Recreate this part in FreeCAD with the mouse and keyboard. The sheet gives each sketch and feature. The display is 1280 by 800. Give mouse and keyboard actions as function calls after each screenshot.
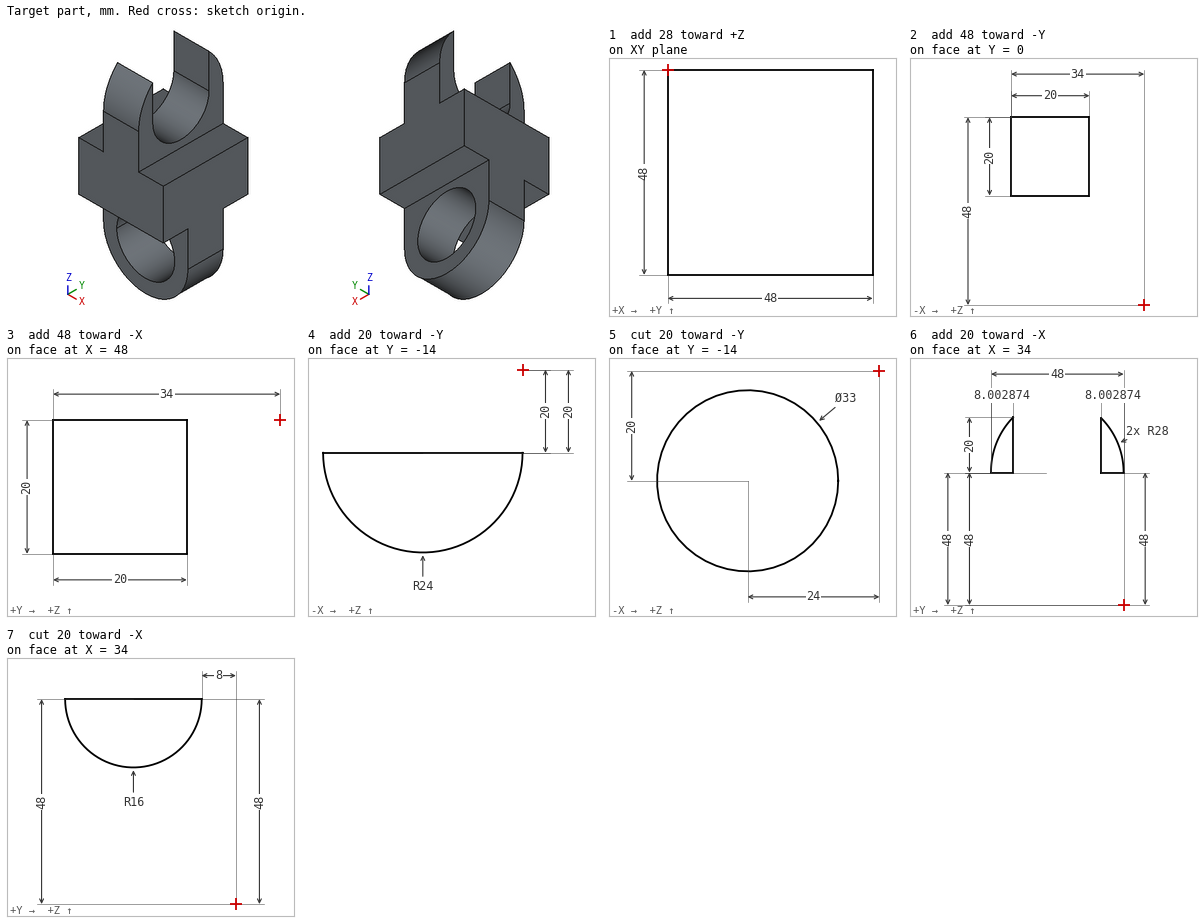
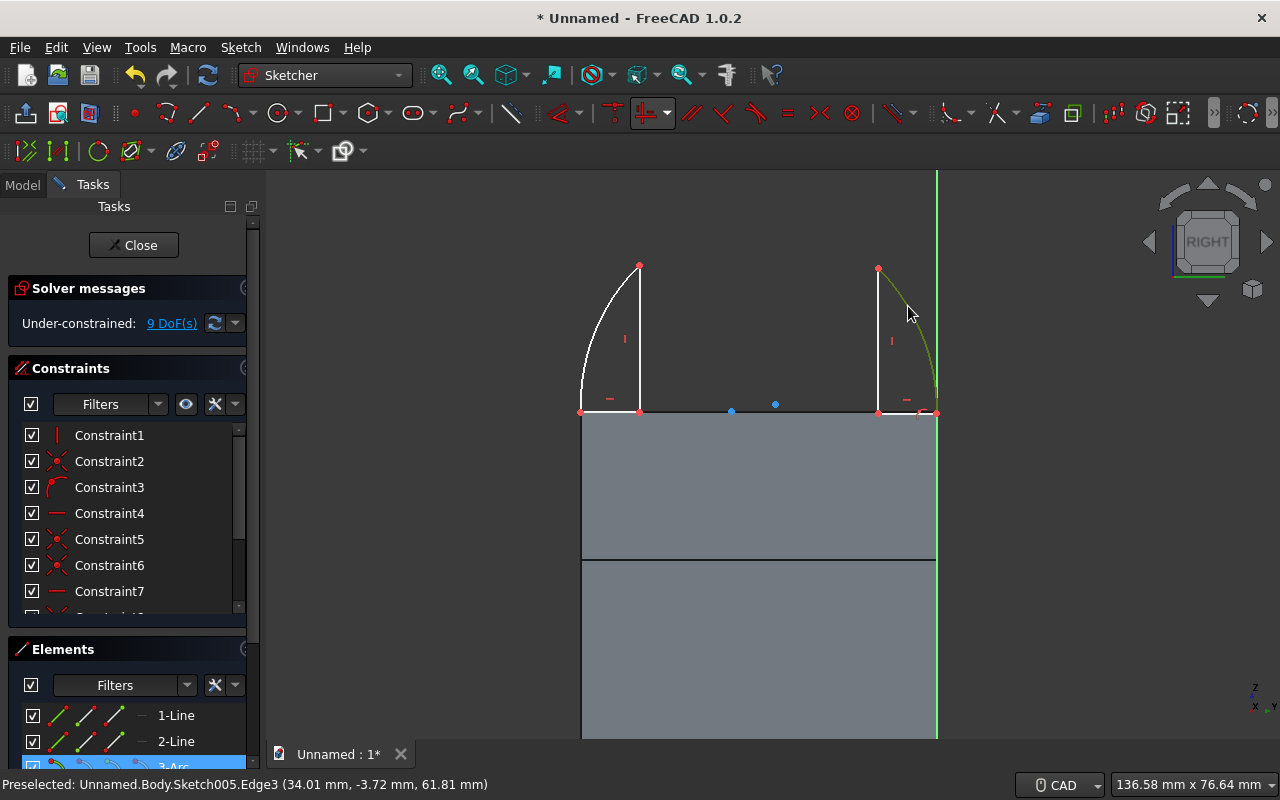
click(609, 303)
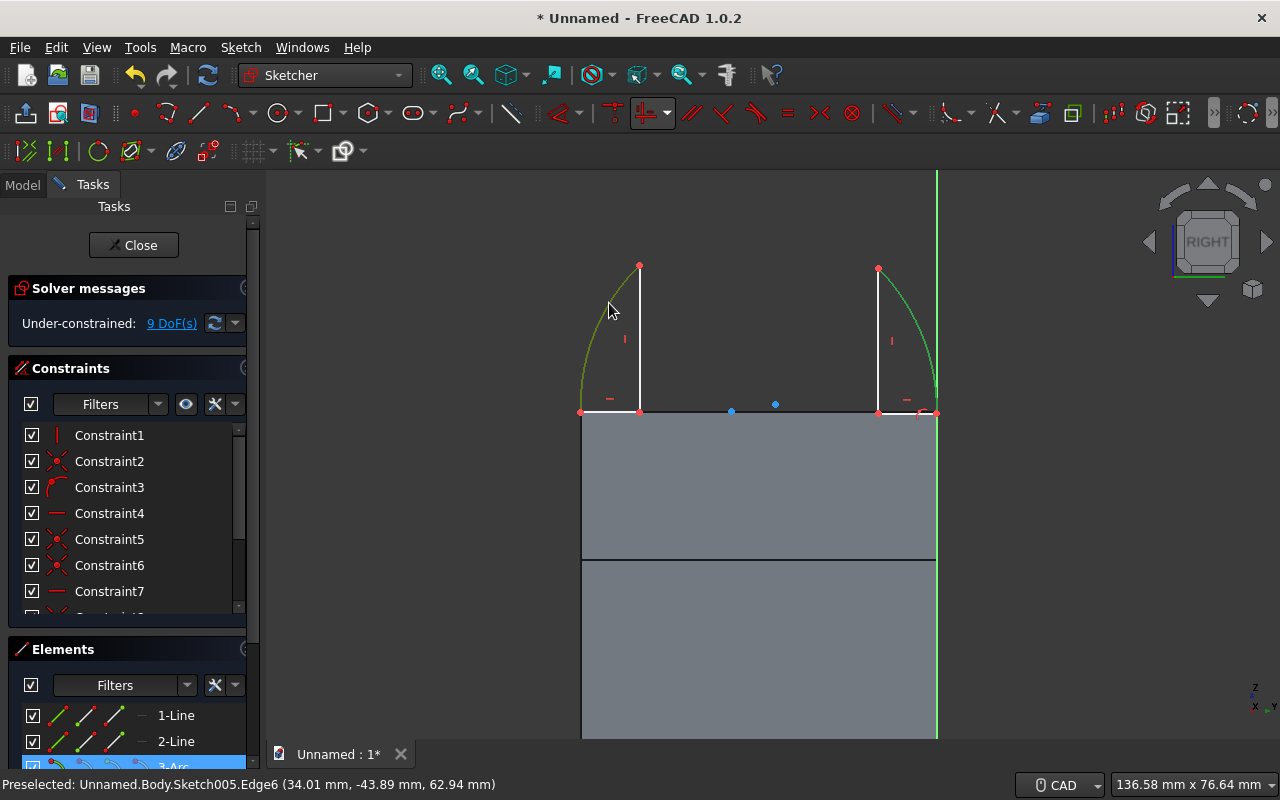
key(e)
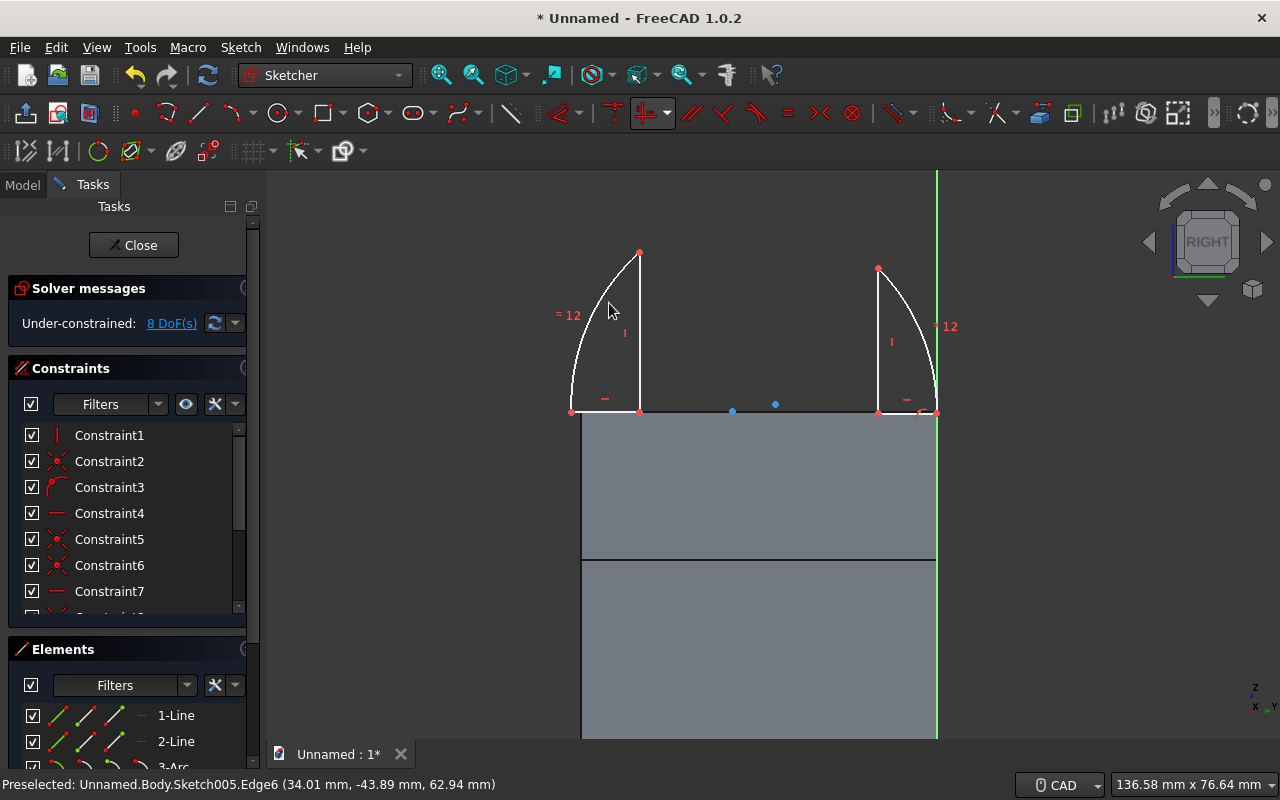
key(d)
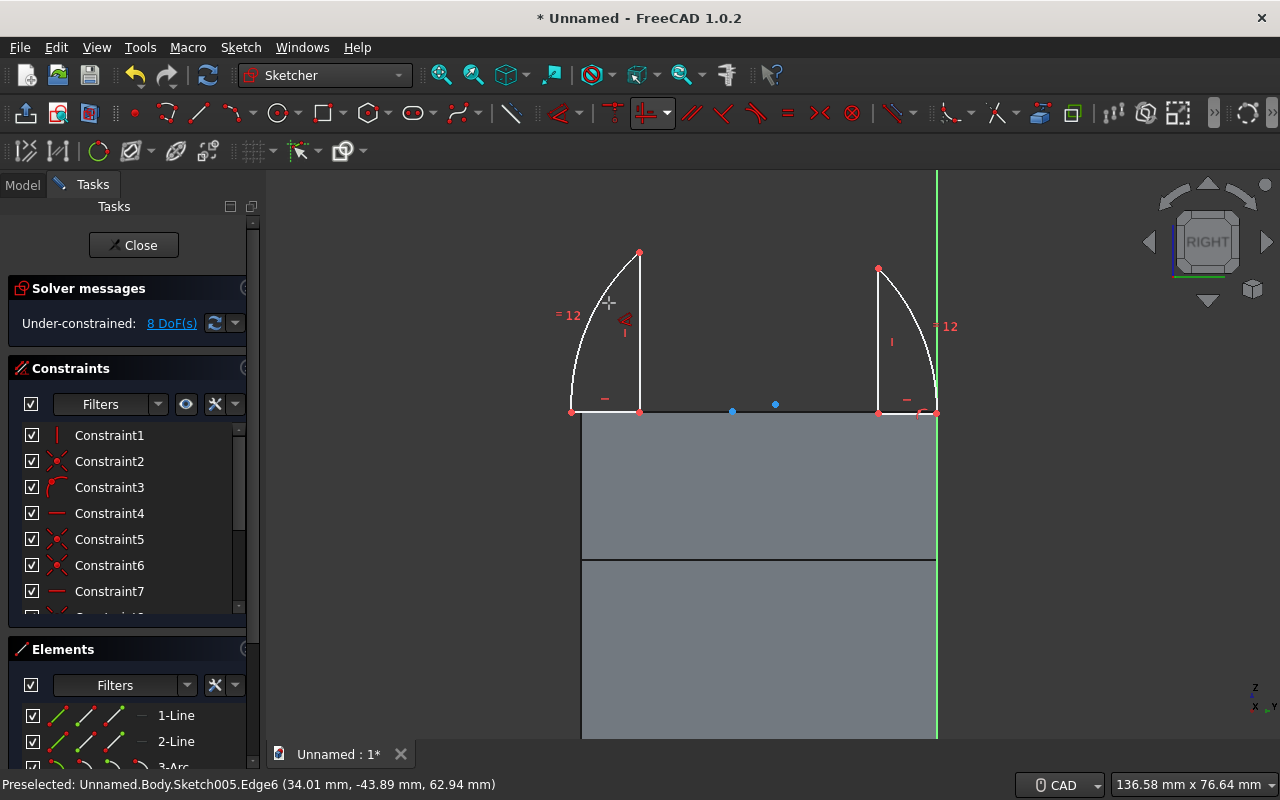
click(908, 306)
click(969, 402)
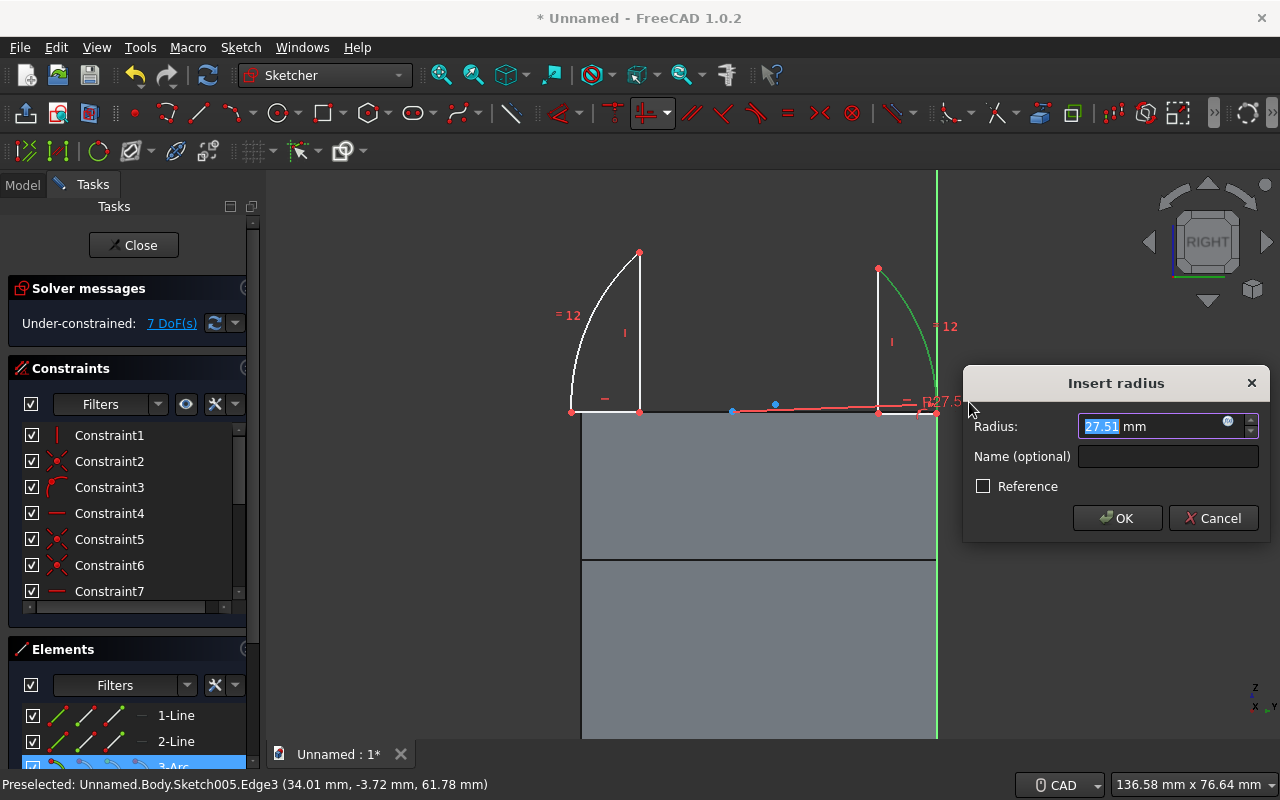
text(28)
key(Return)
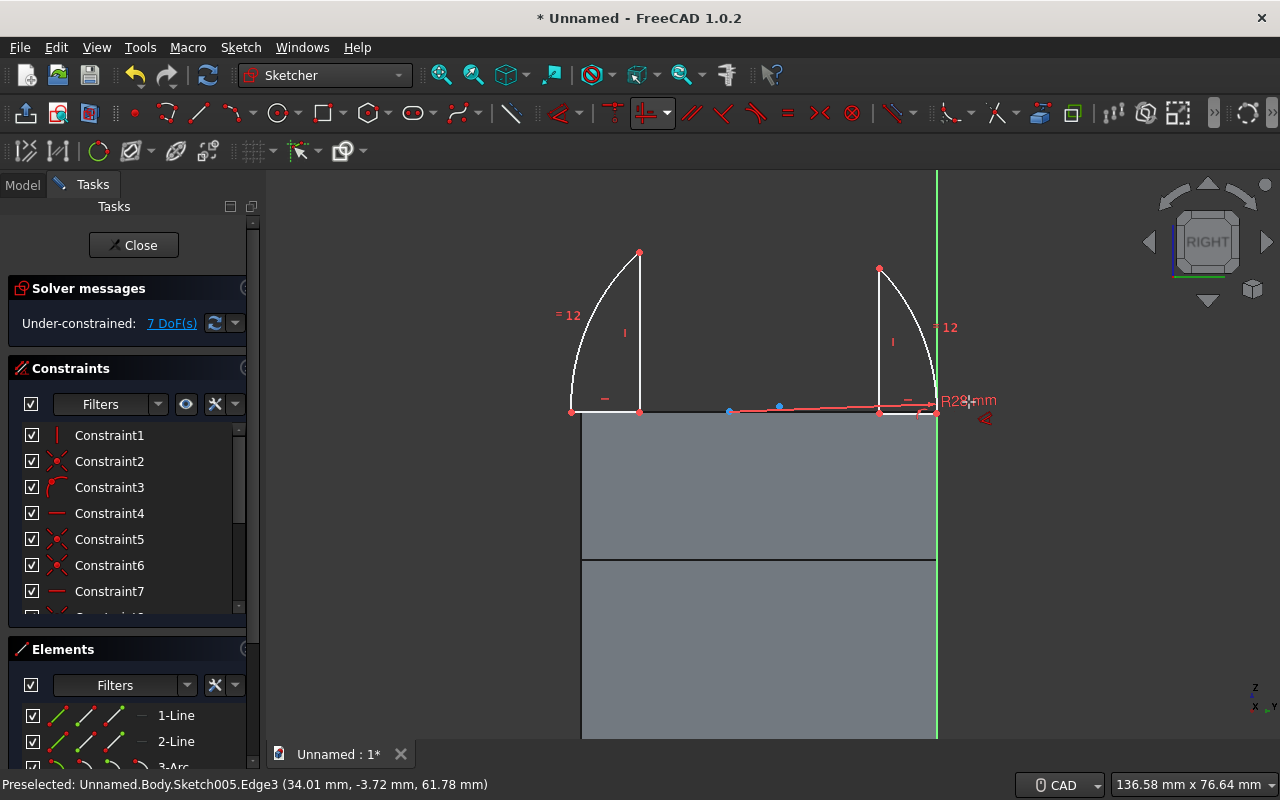
click(640, 364)
click(606, 332)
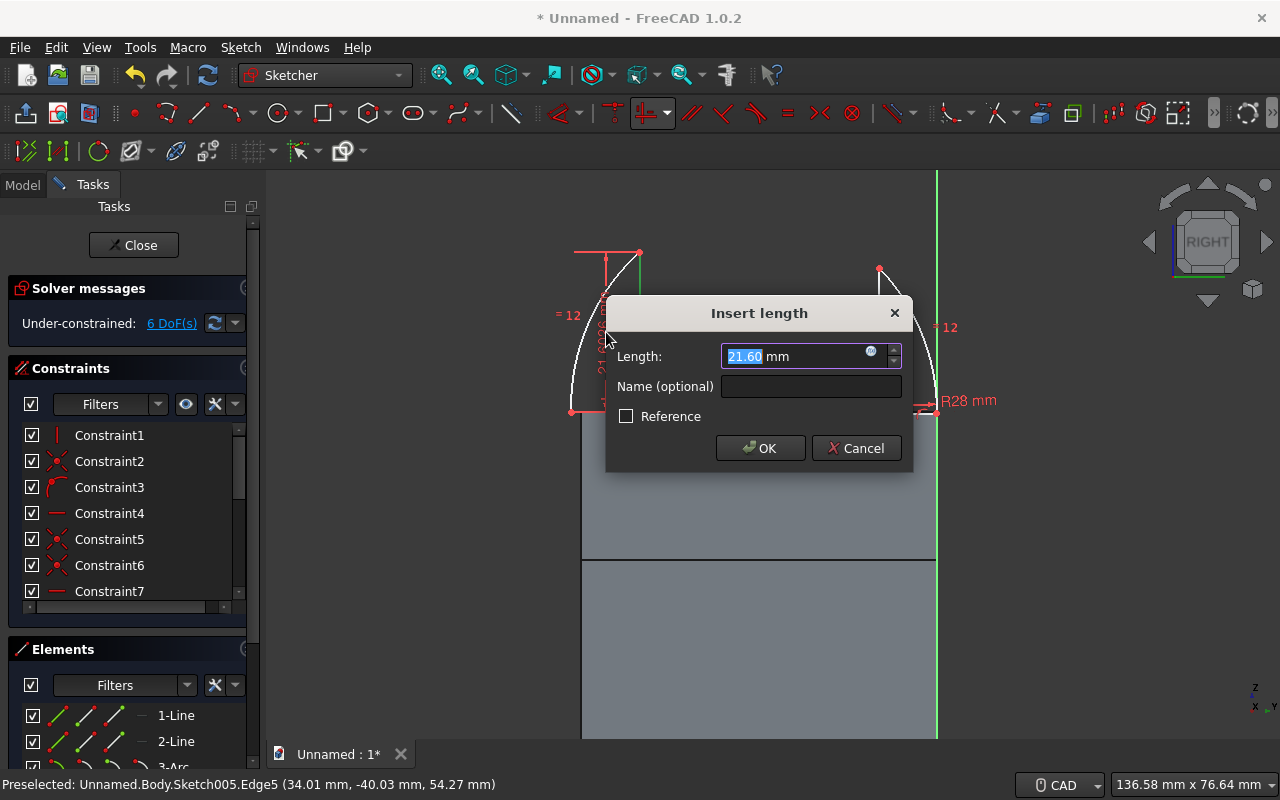
text(20)
key(Return)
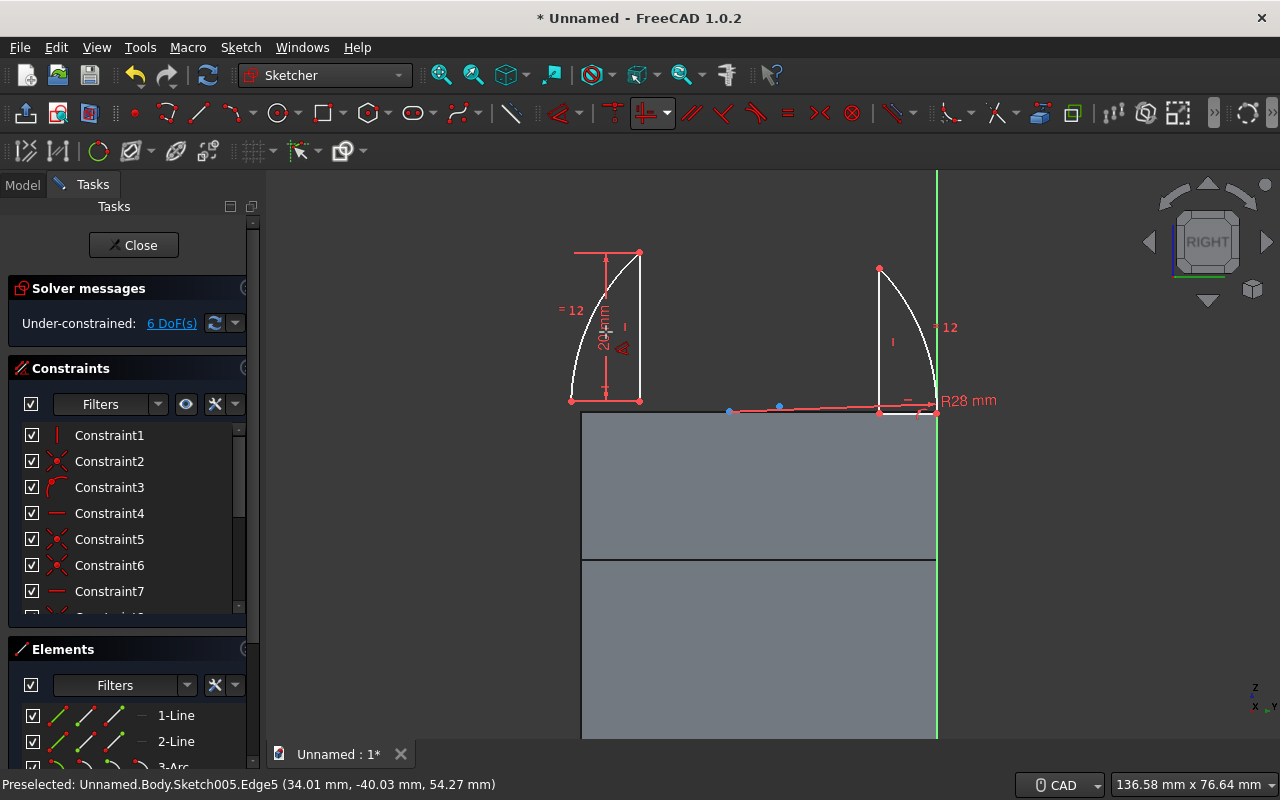
click(879, 414)
click(971, 562)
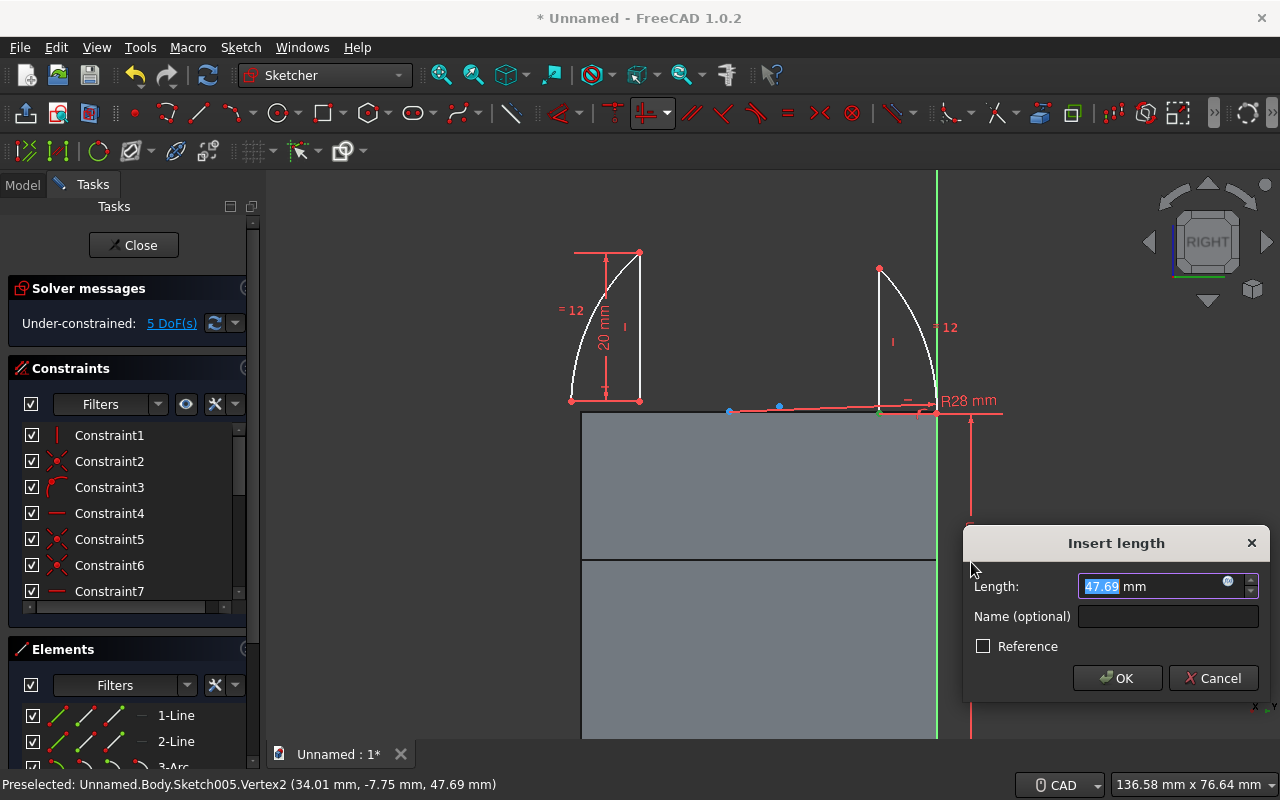
text(48)
key(Return)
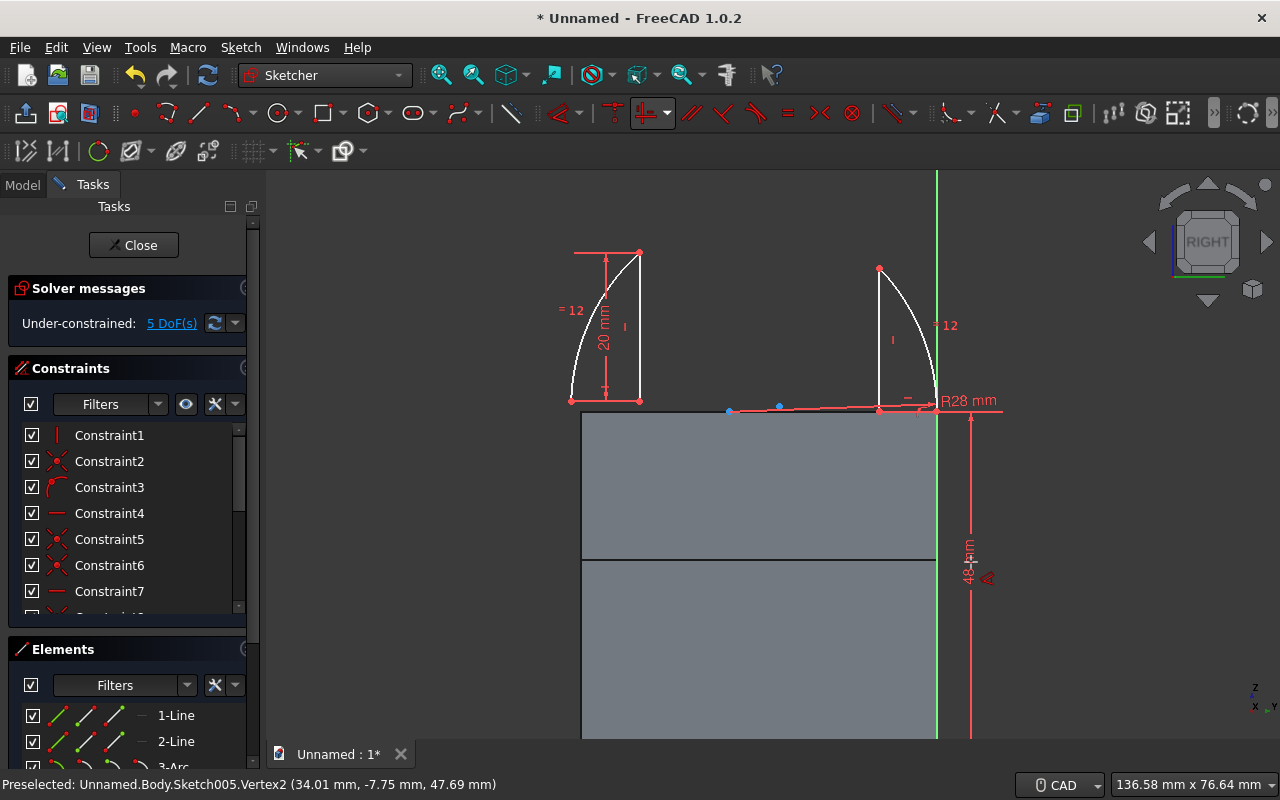
click(571, 401)
click(754, 367)